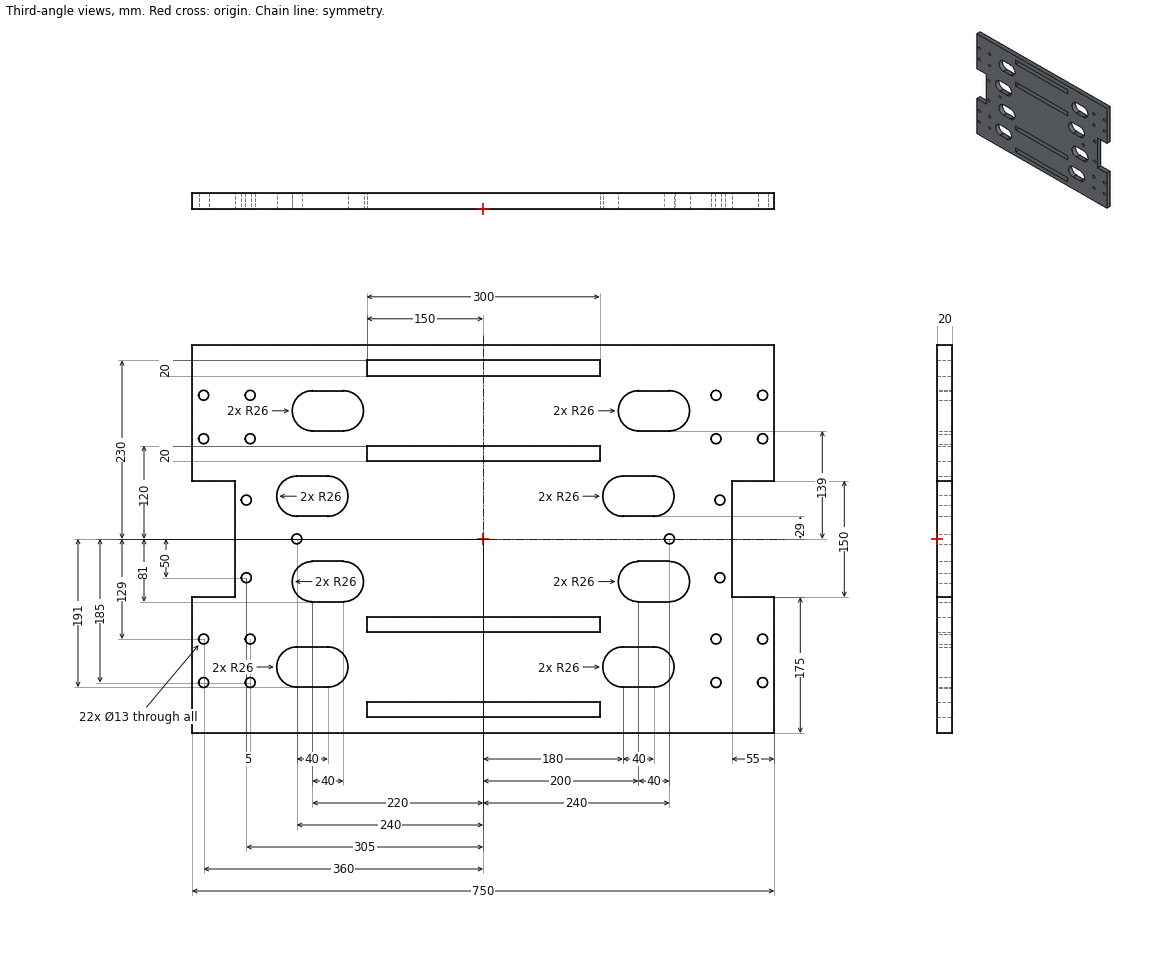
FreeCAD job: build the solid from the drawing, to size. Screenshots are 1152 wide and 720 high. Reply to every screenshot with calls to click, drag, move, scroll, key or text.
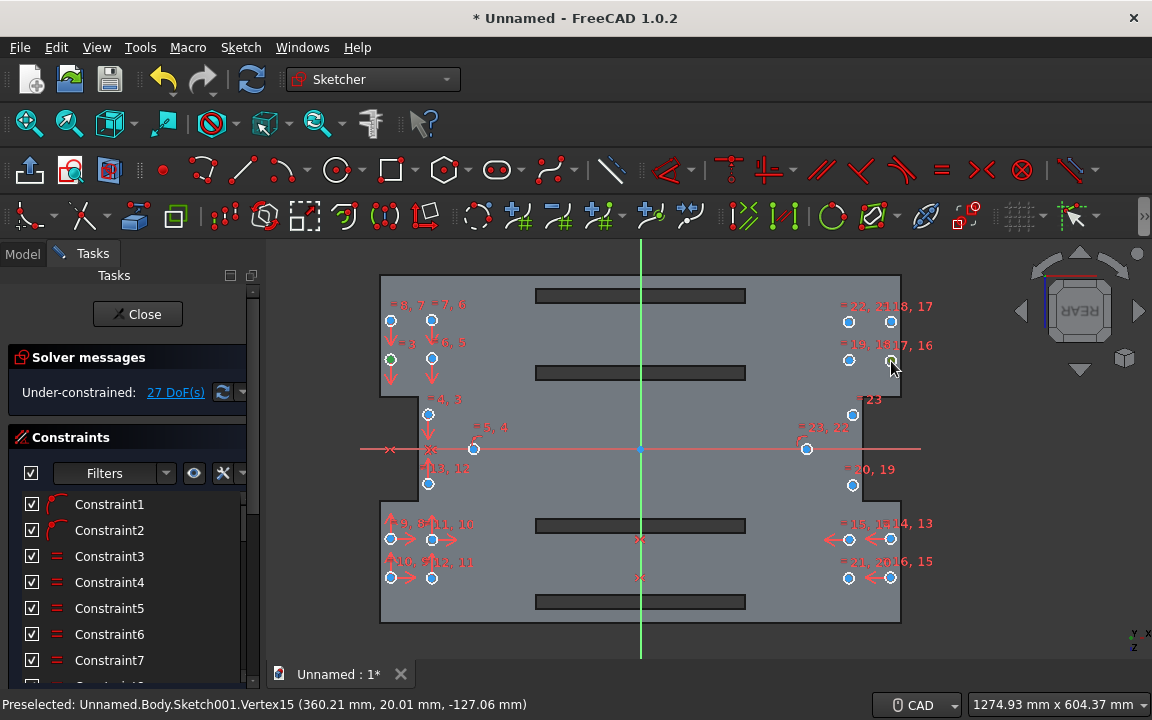
click(641, 605)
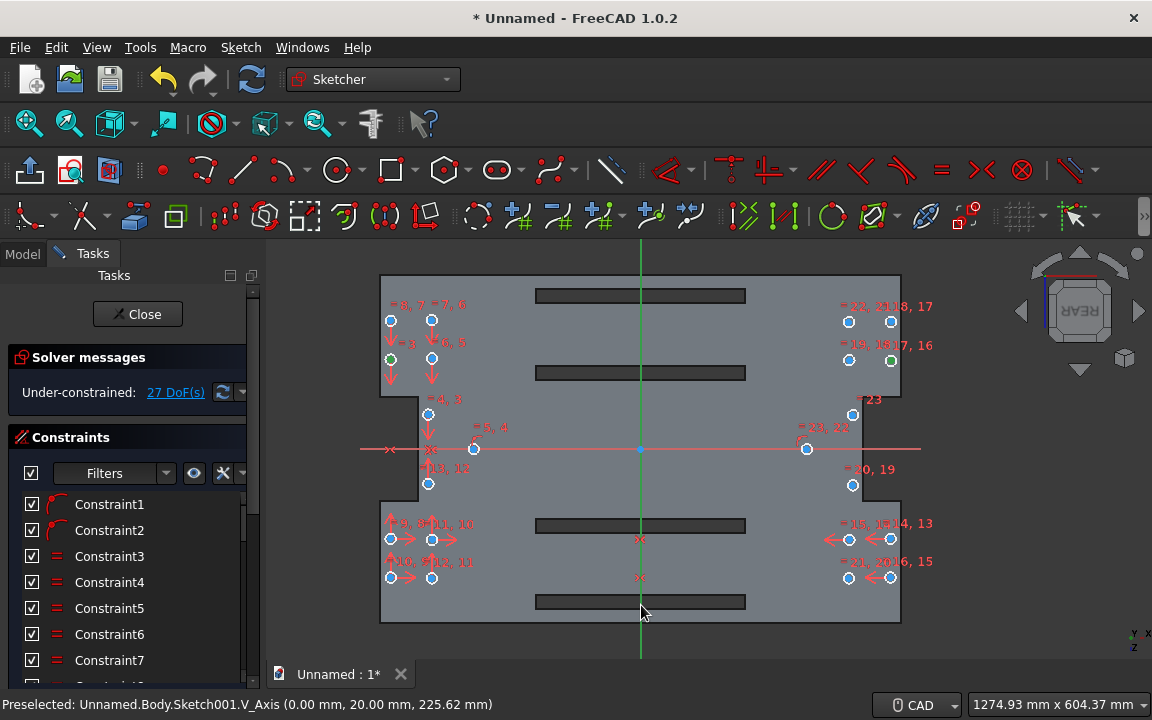
click(982, 170)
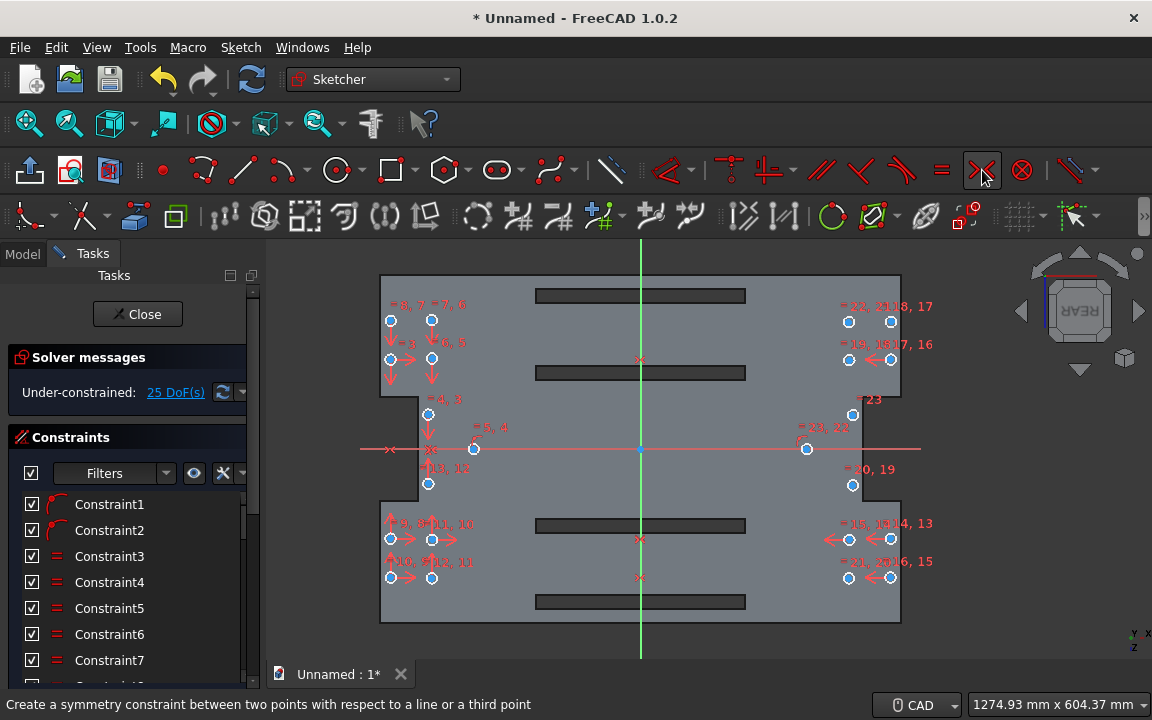
click(391, 321)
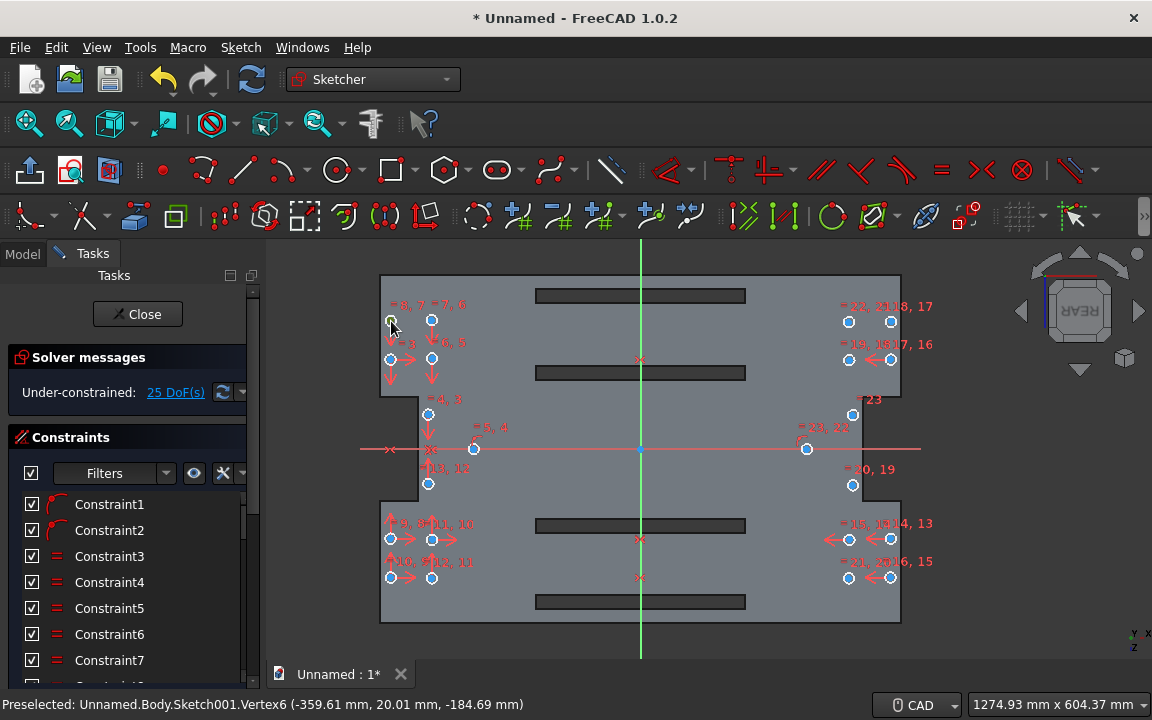
click(891, 322)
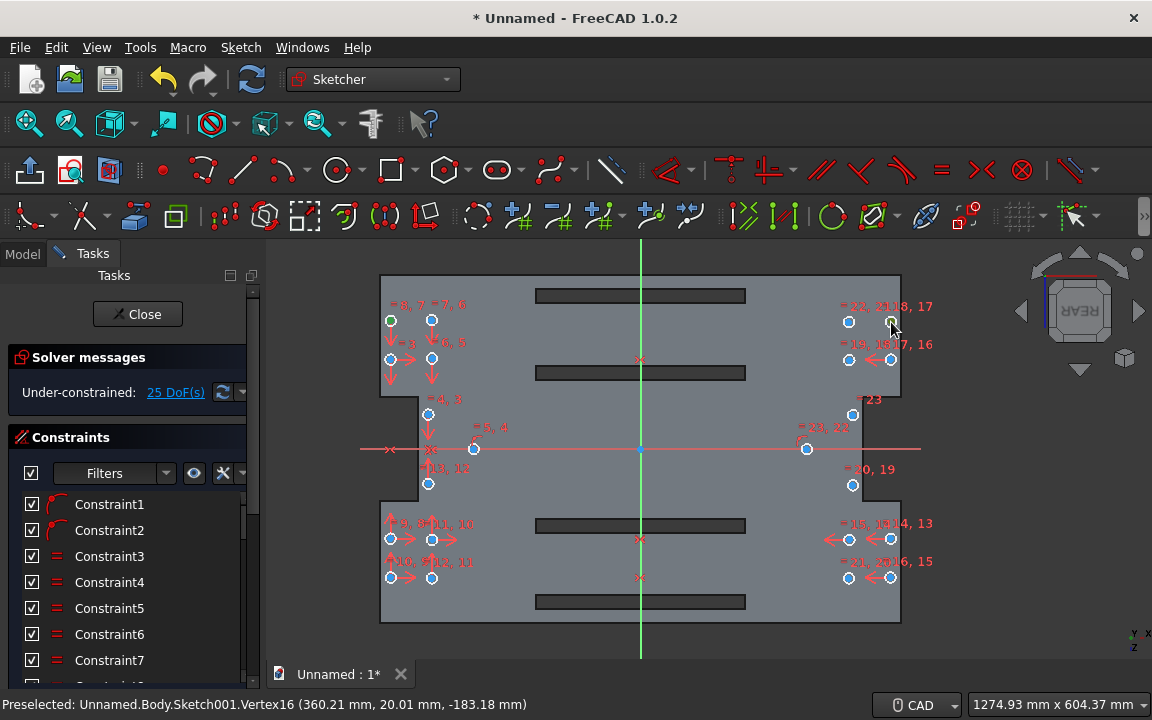
click(641, 605)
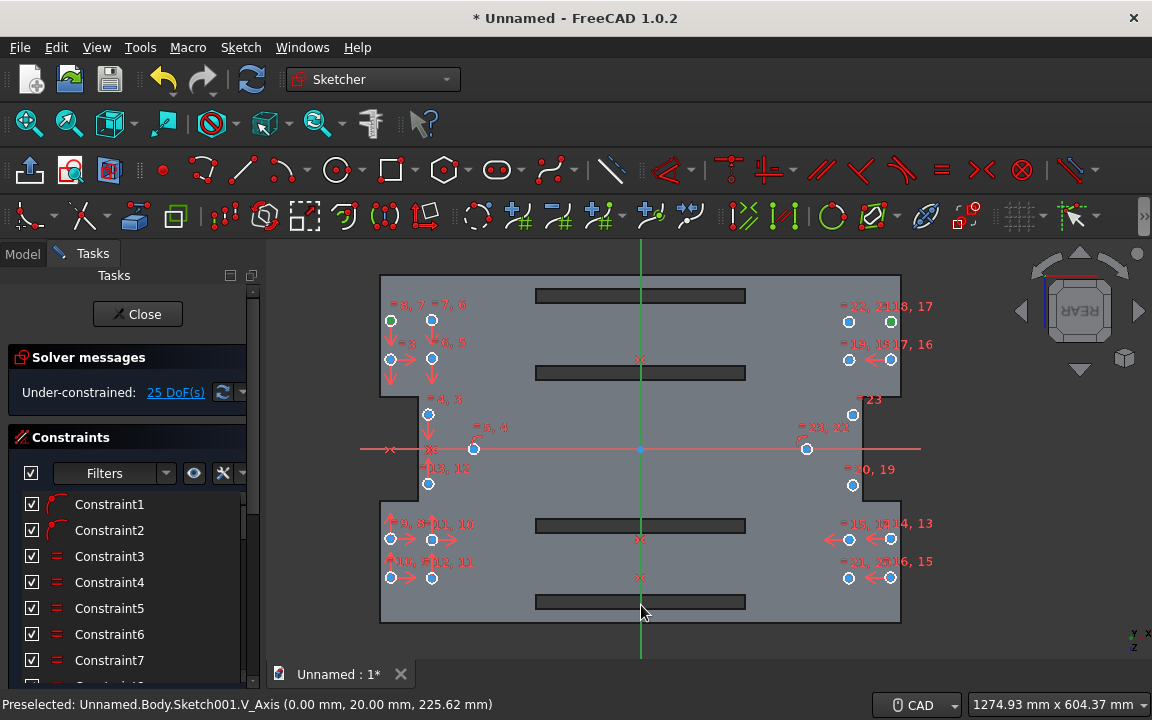
click(982, 170)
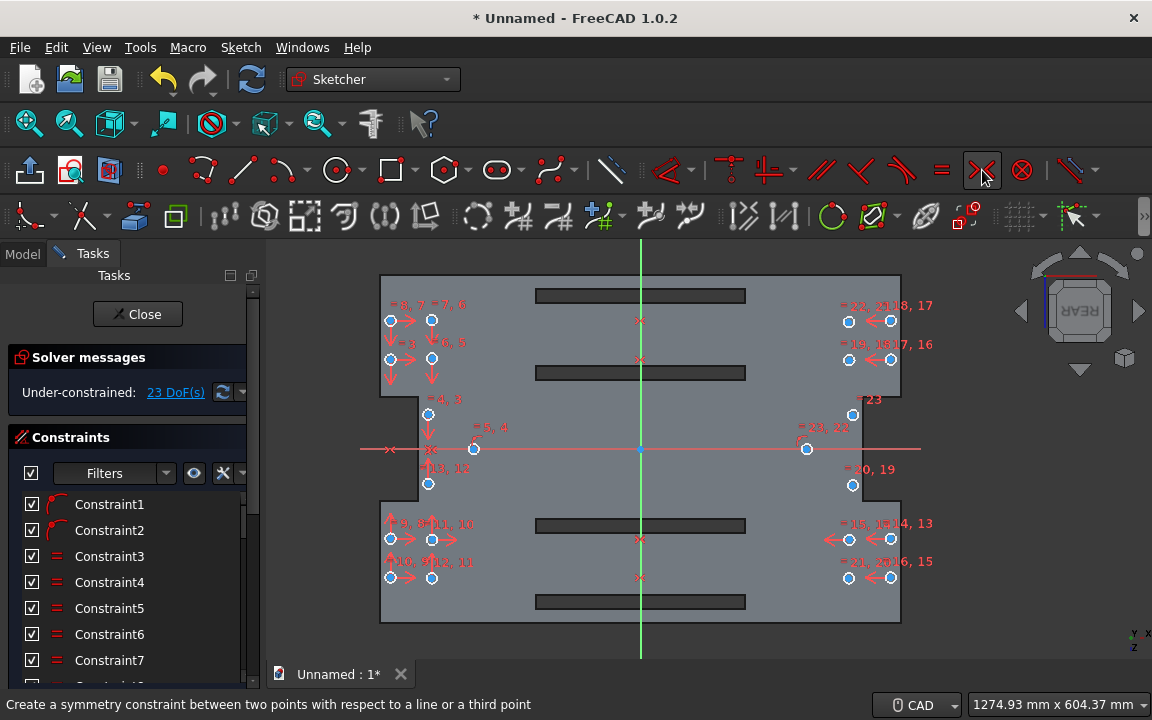
click(432, 359)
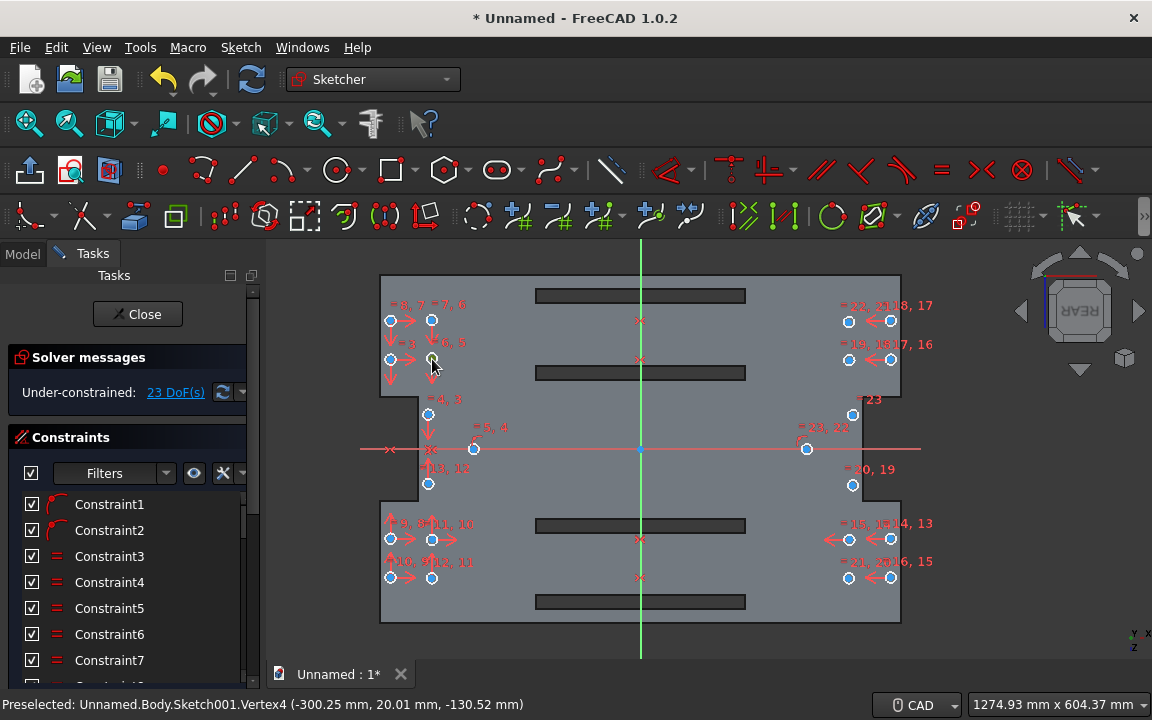
click(849, 360)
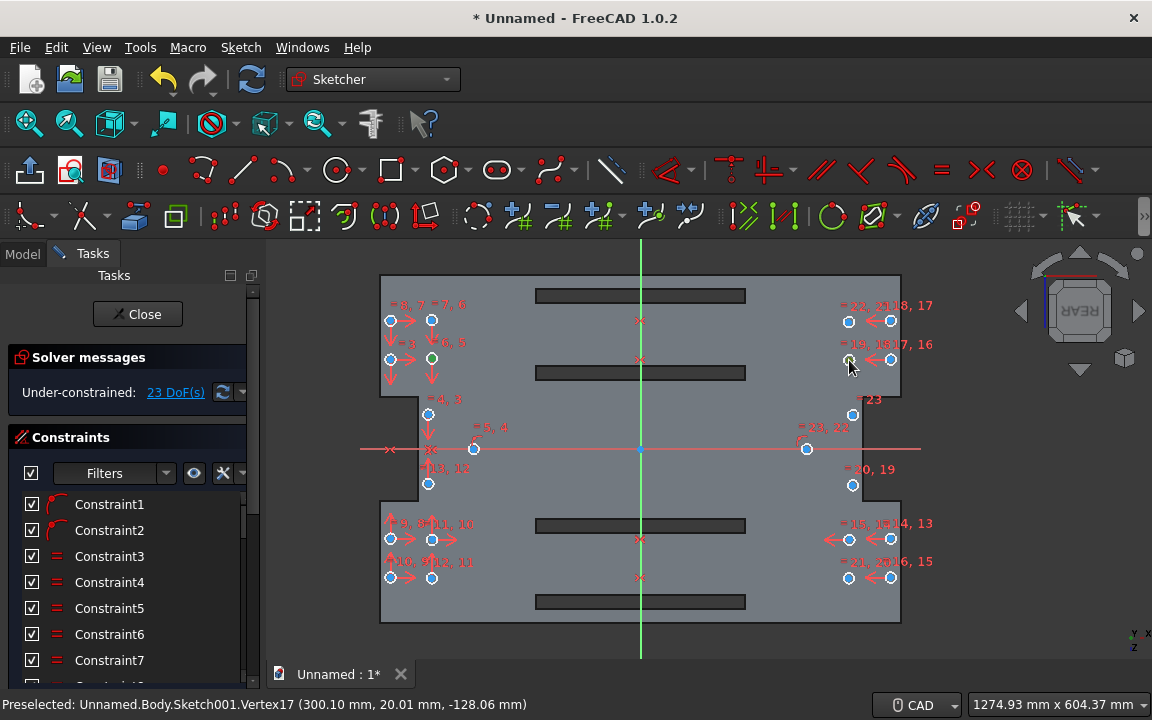
click(641, 605)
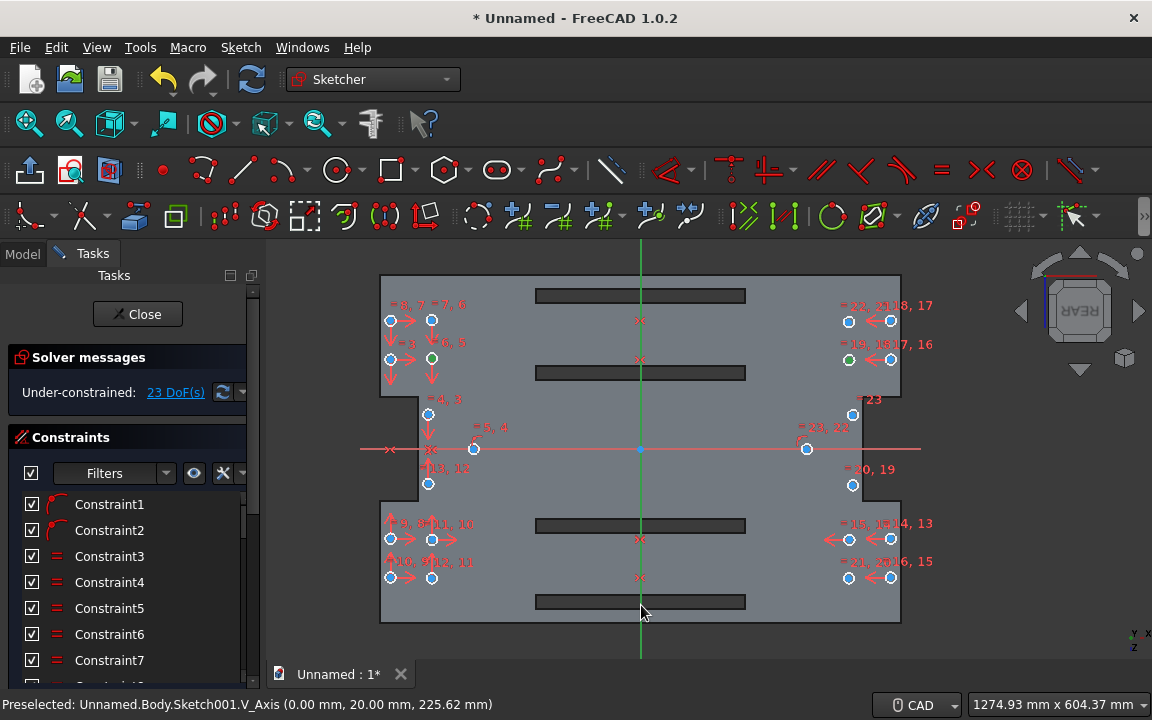
click(982, 170)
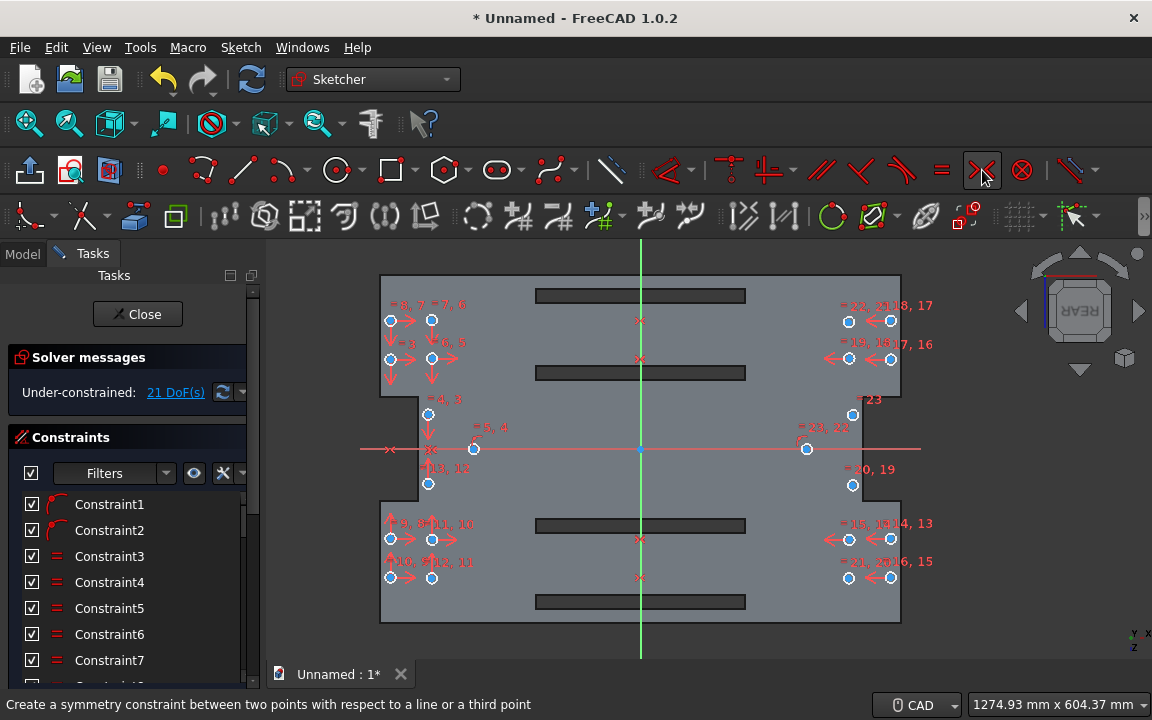
click(428, 484)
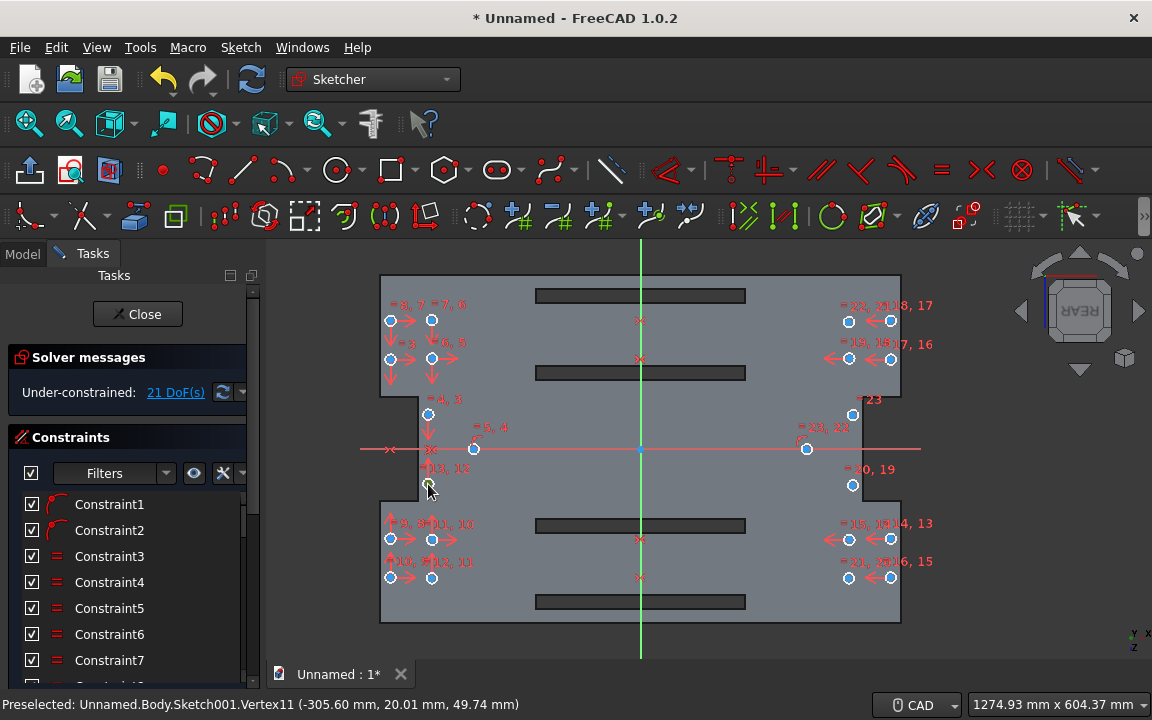
click(853, 485)